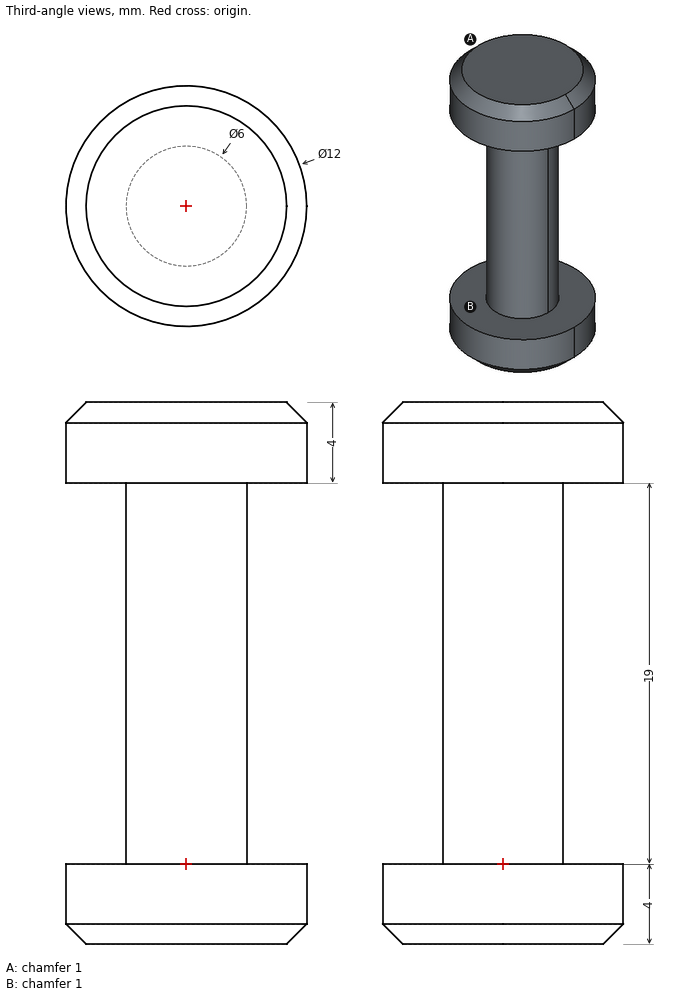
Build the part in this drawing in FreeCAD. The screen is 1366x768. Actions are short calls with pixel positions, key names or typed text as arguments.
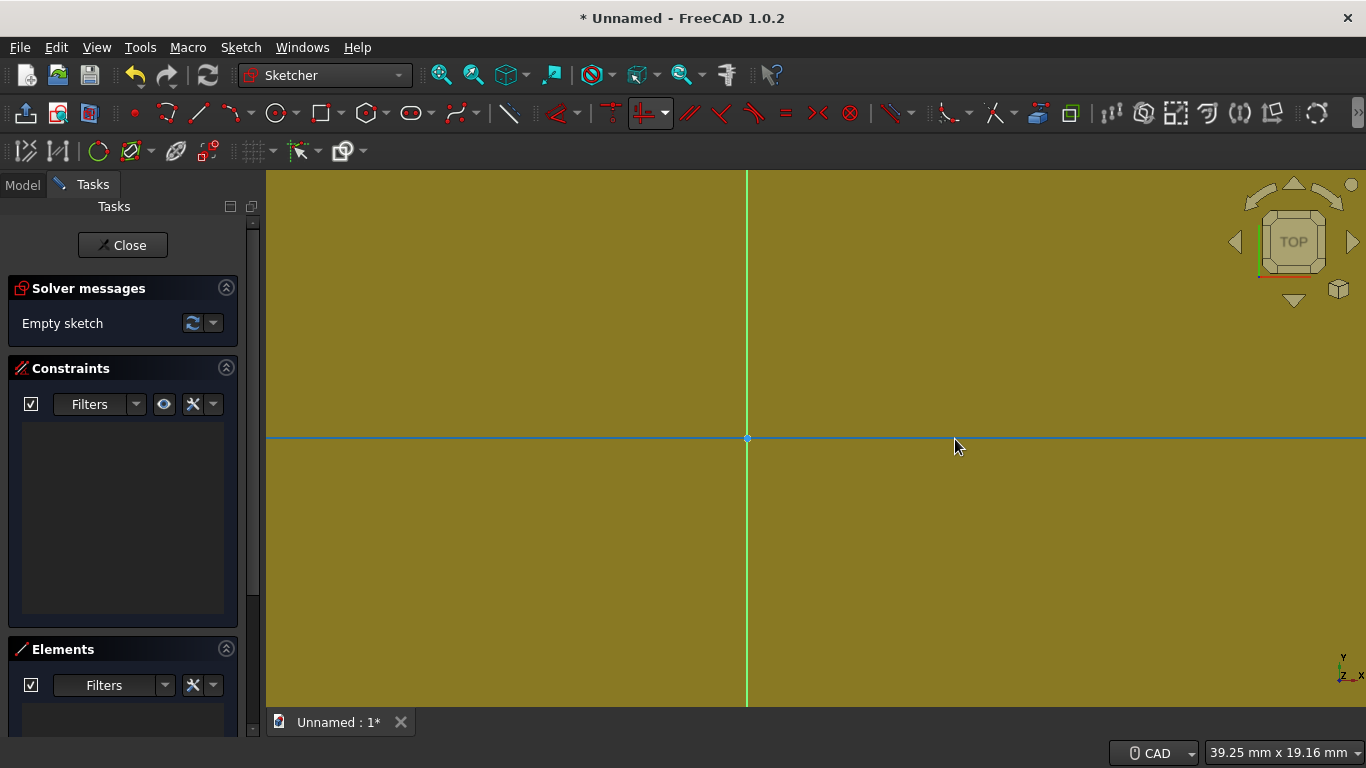
key(g)
key(c)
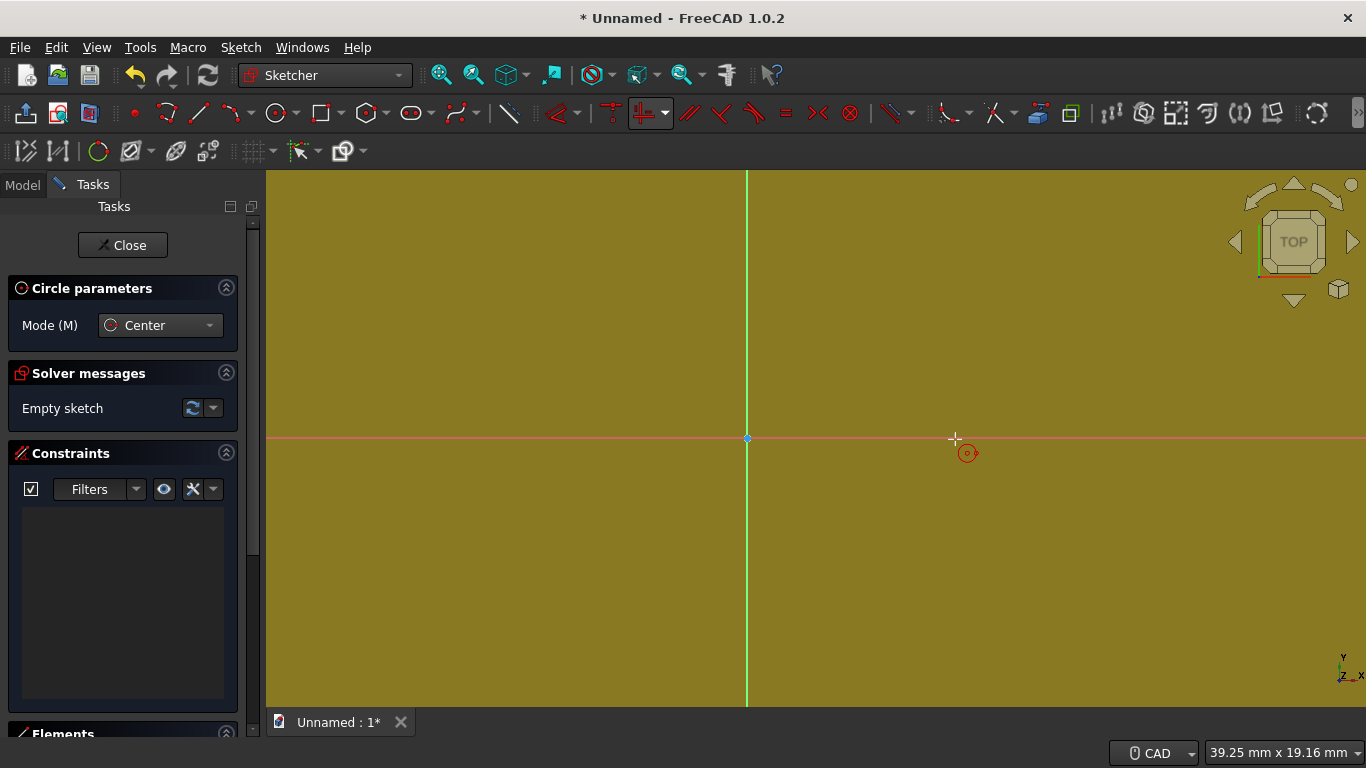
click(747, 438)
move(866, 319)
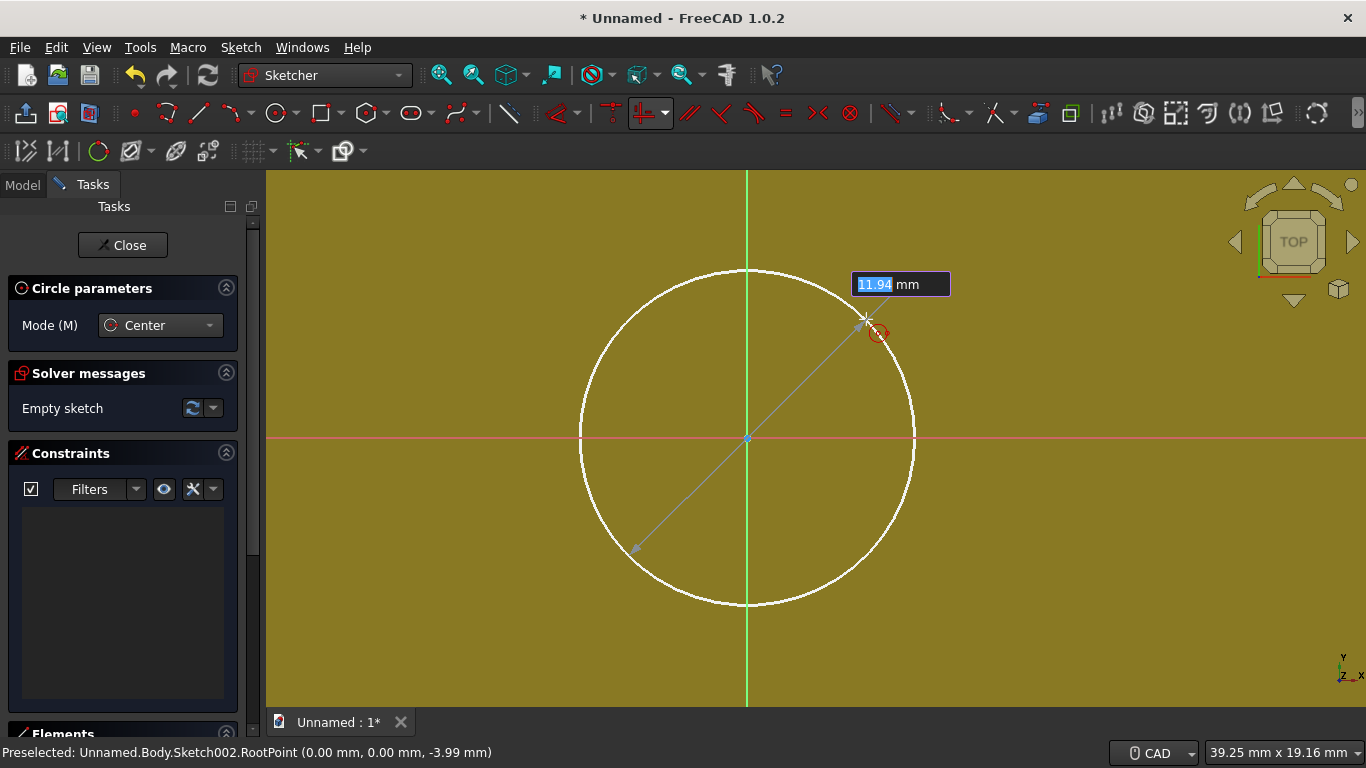
text(12)
key(Return)
key(Escape)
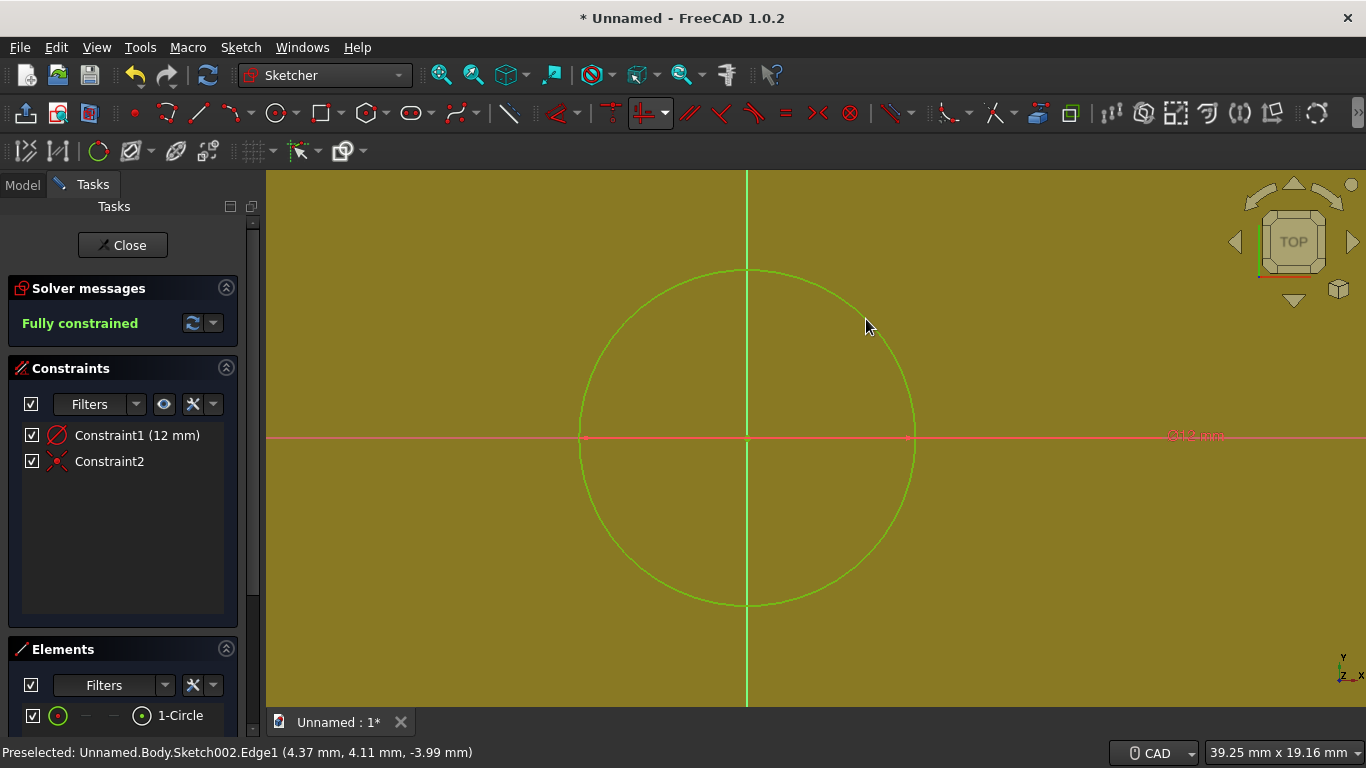
click(123, 245)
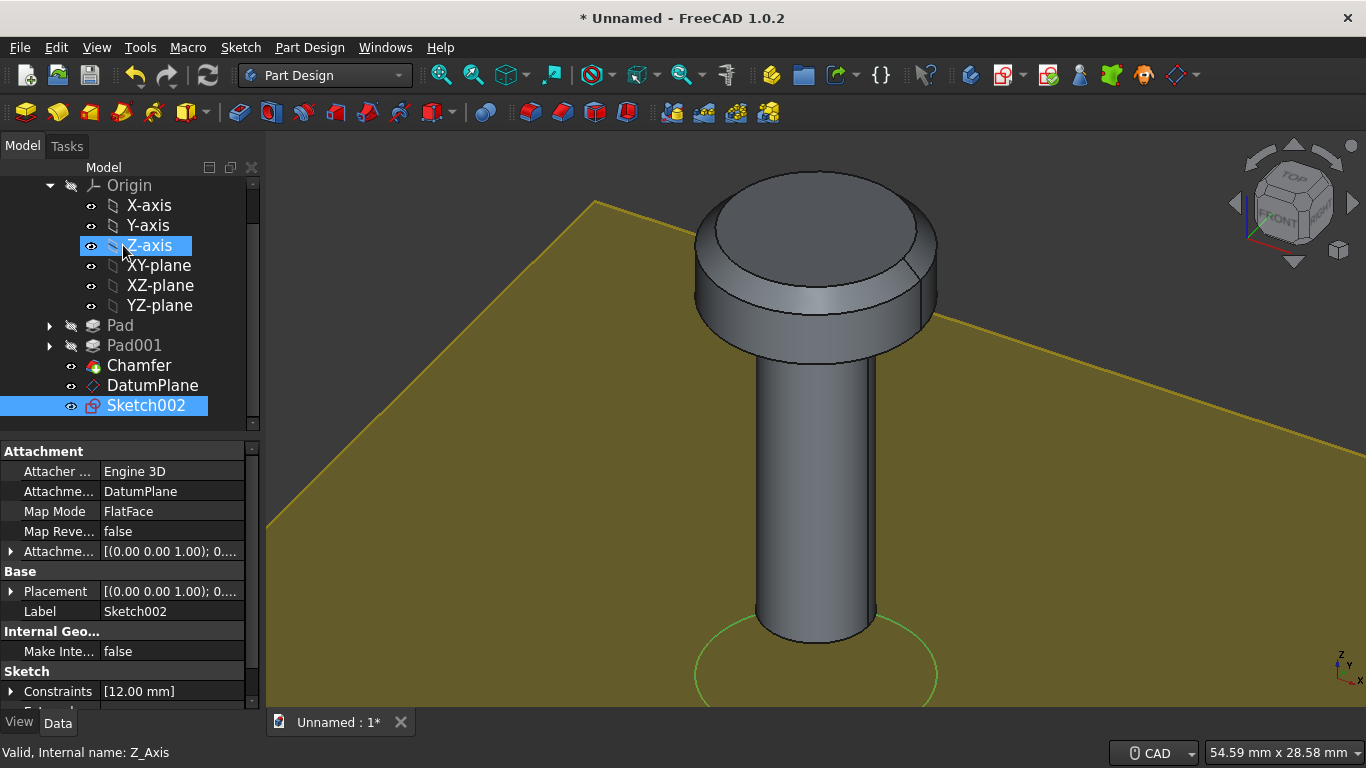
click(26, 112)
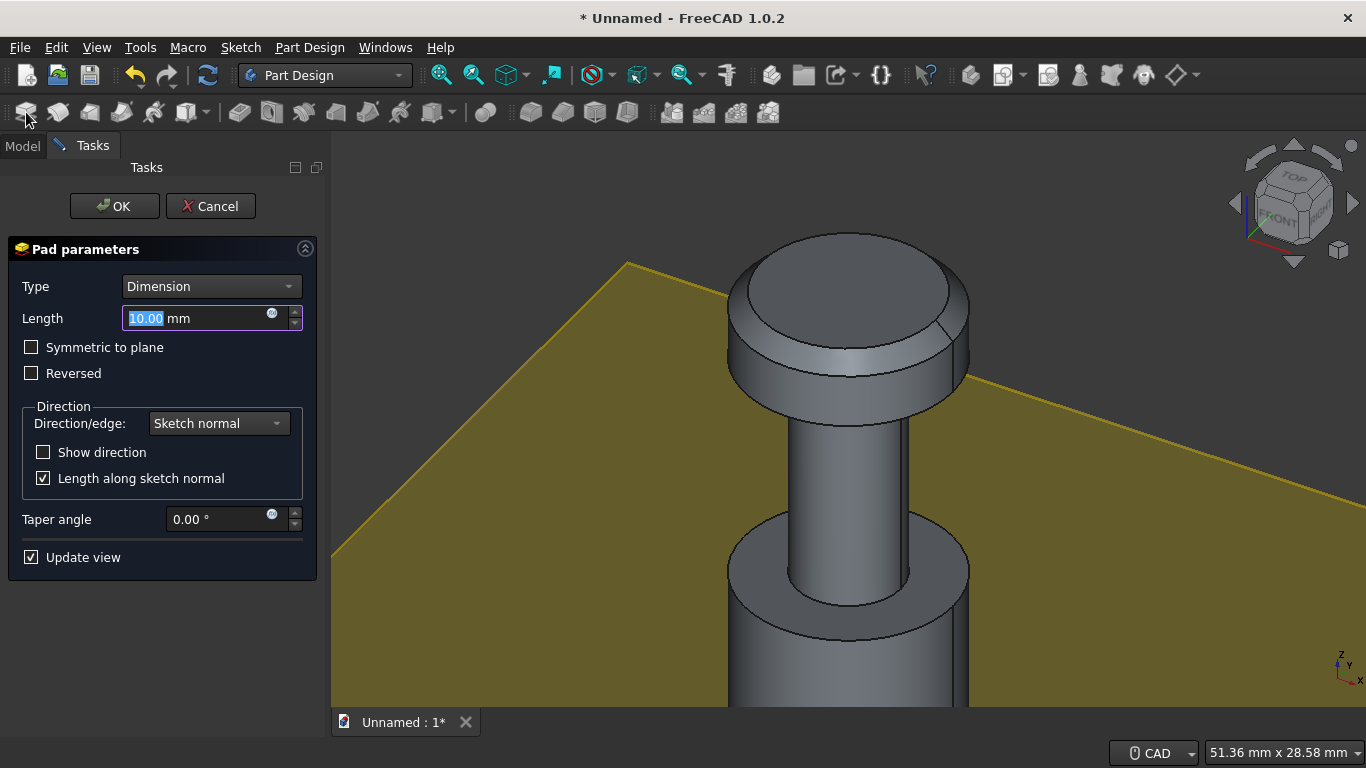
text(4)
key(Tab)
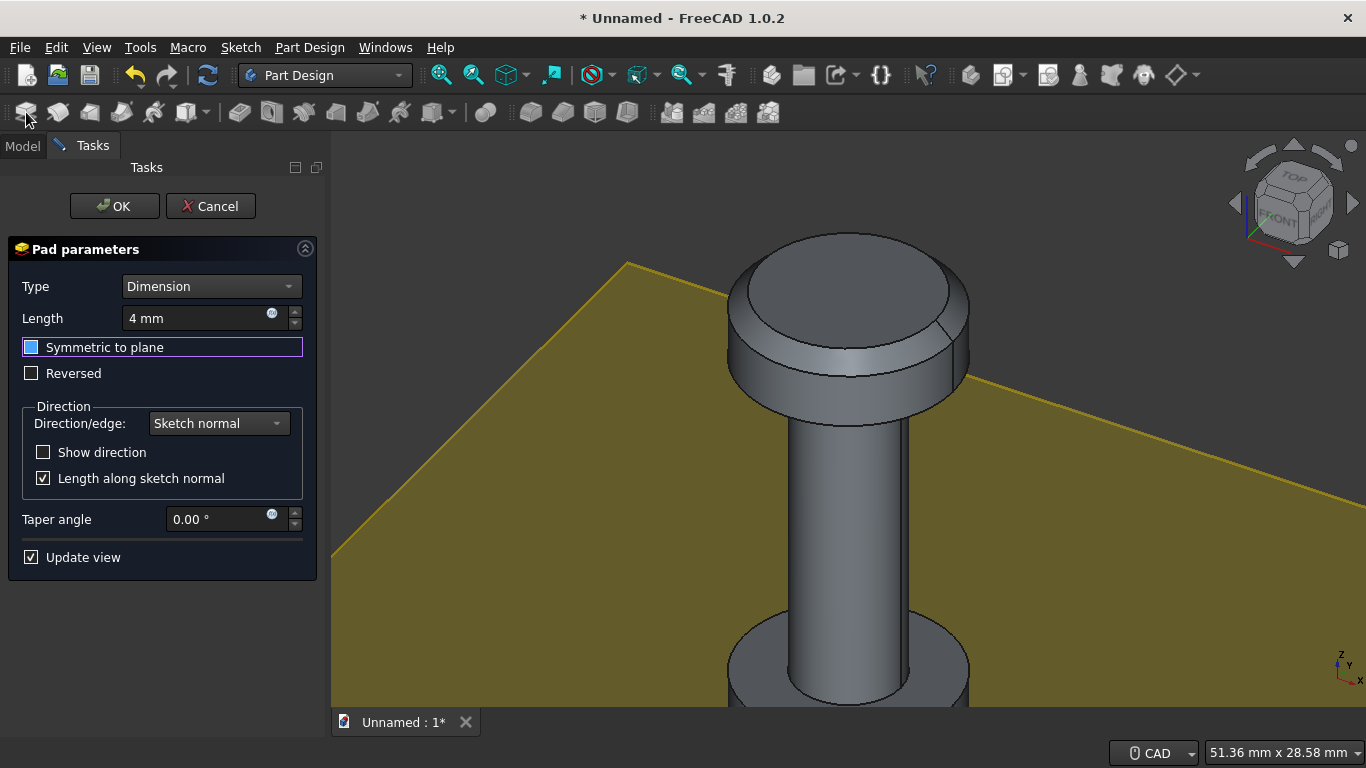
click(115, 206)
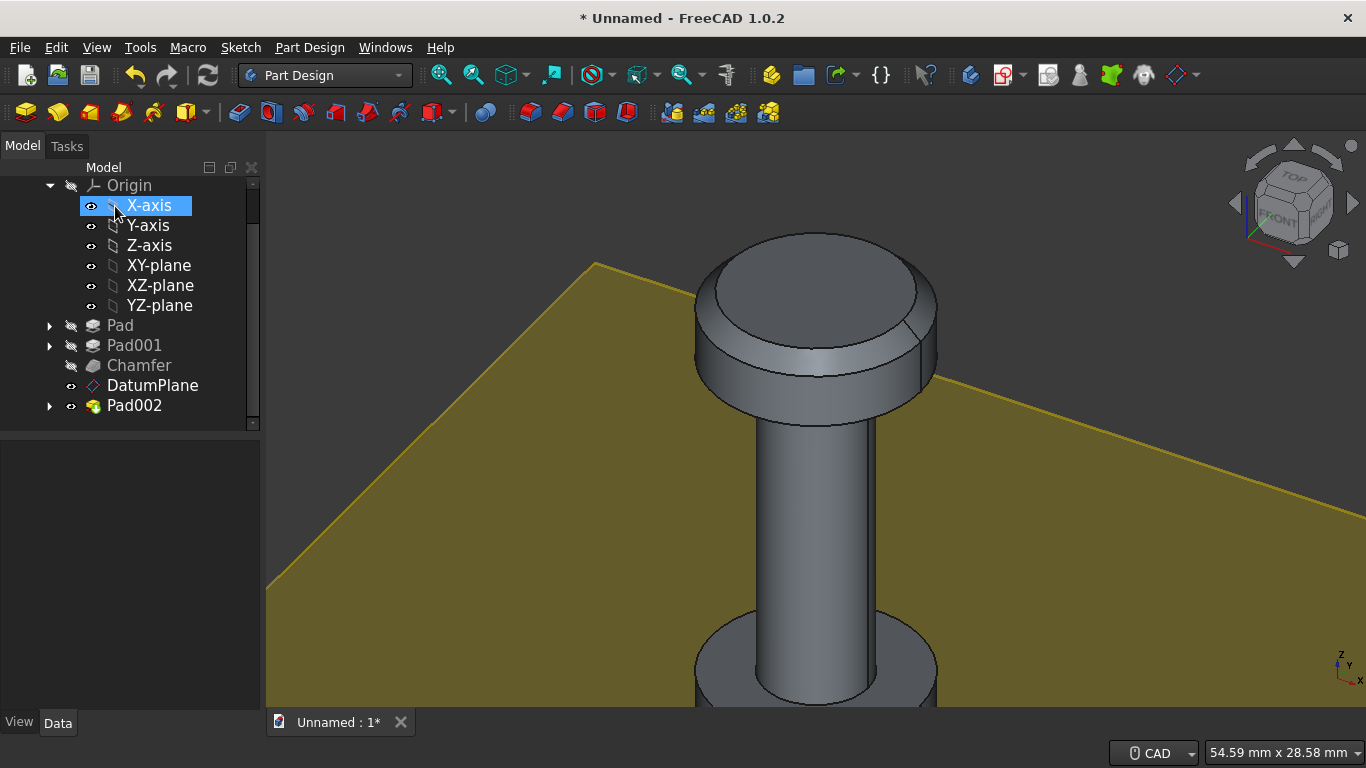
click(116, 386)
key(space)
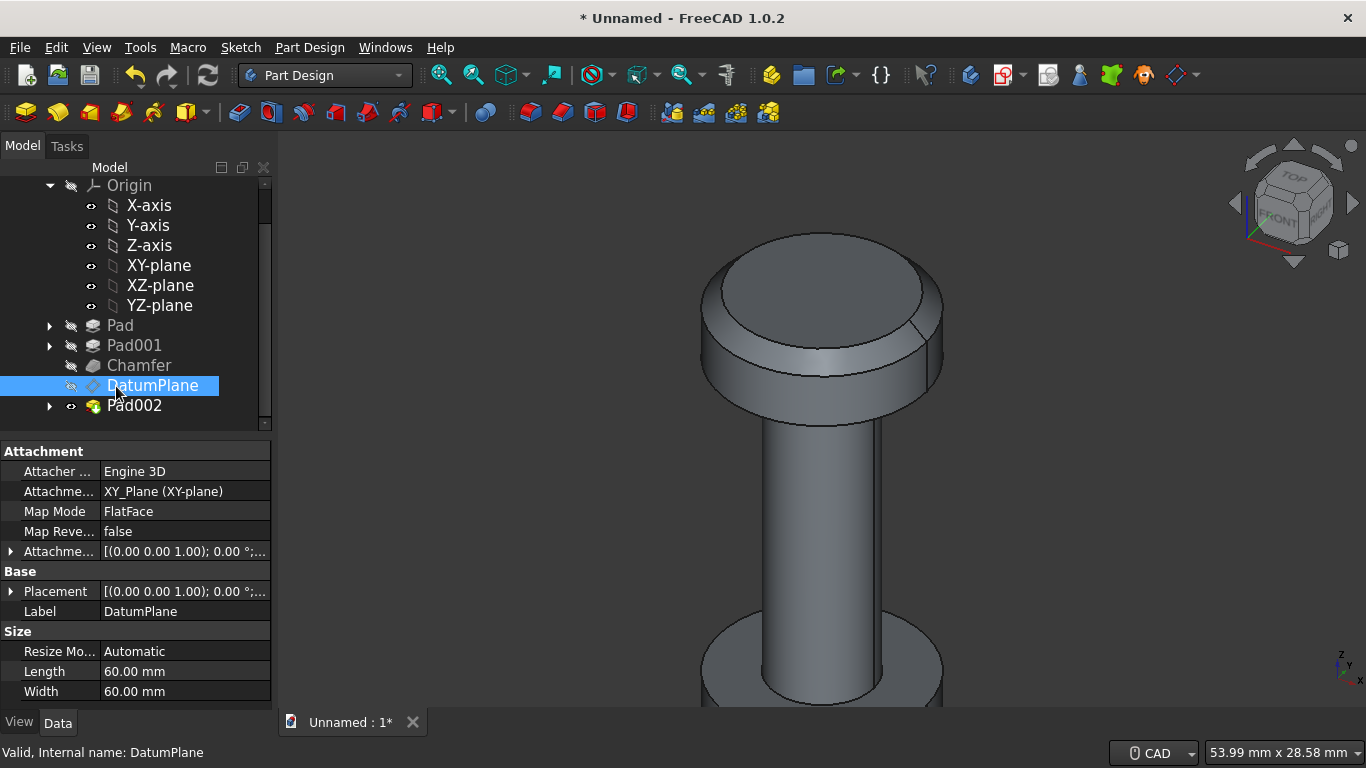
key(v)
key(f)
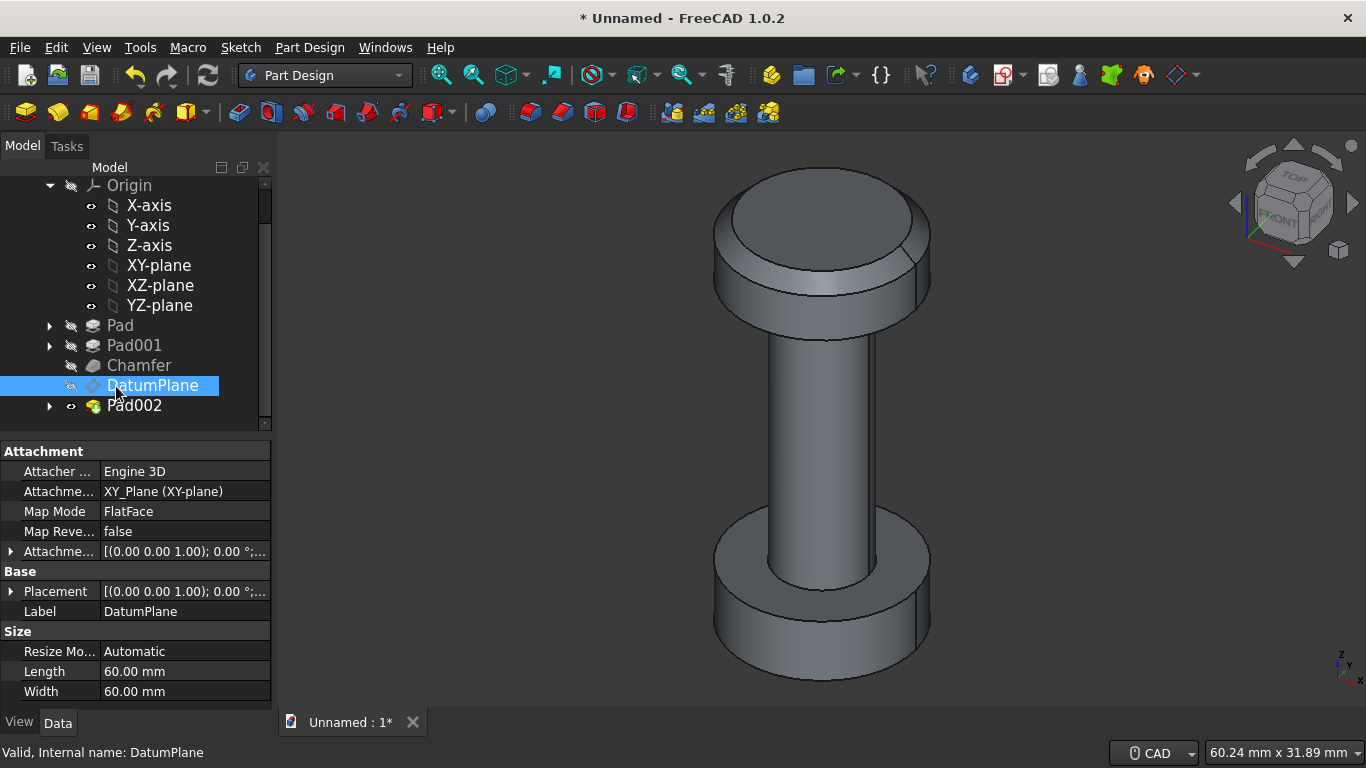
key(0)